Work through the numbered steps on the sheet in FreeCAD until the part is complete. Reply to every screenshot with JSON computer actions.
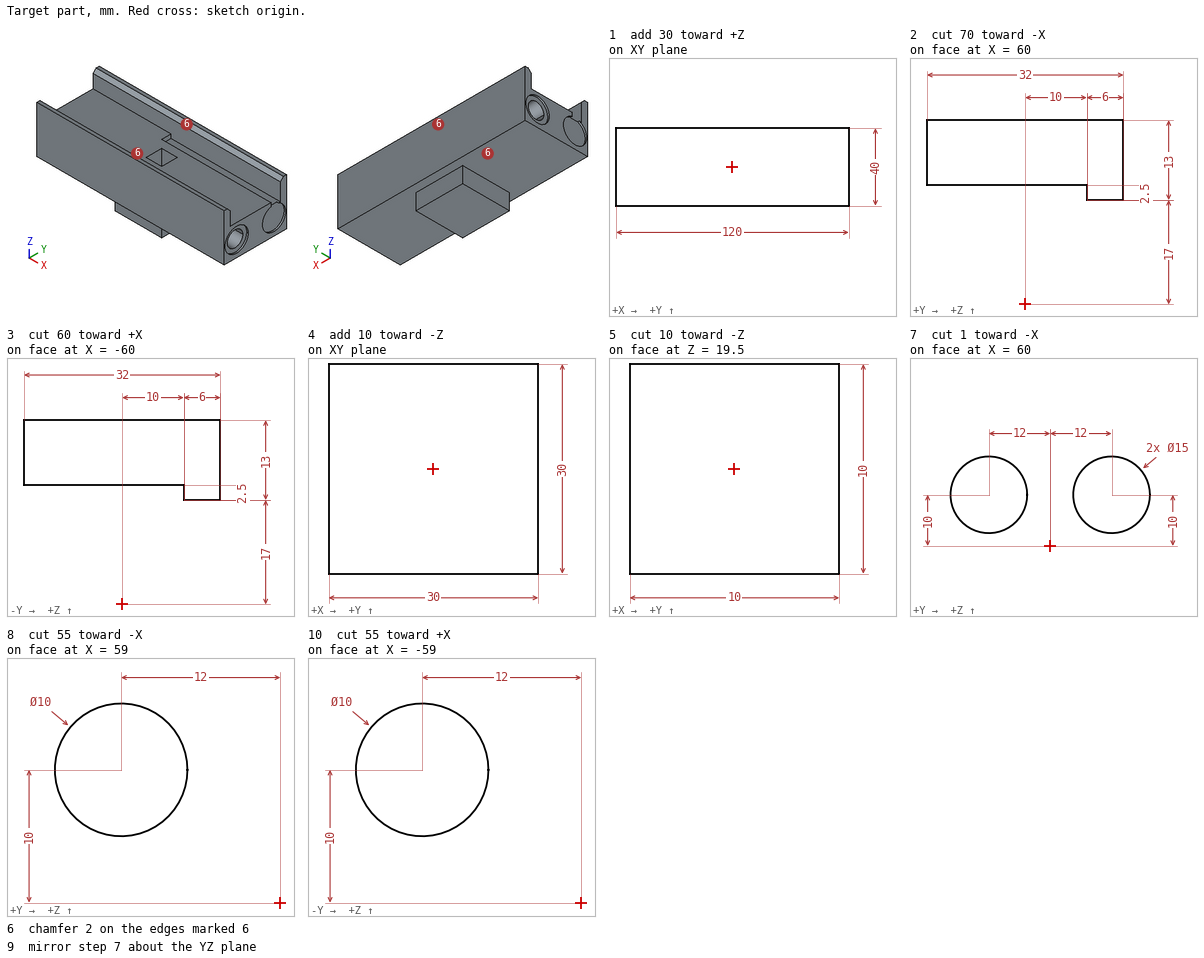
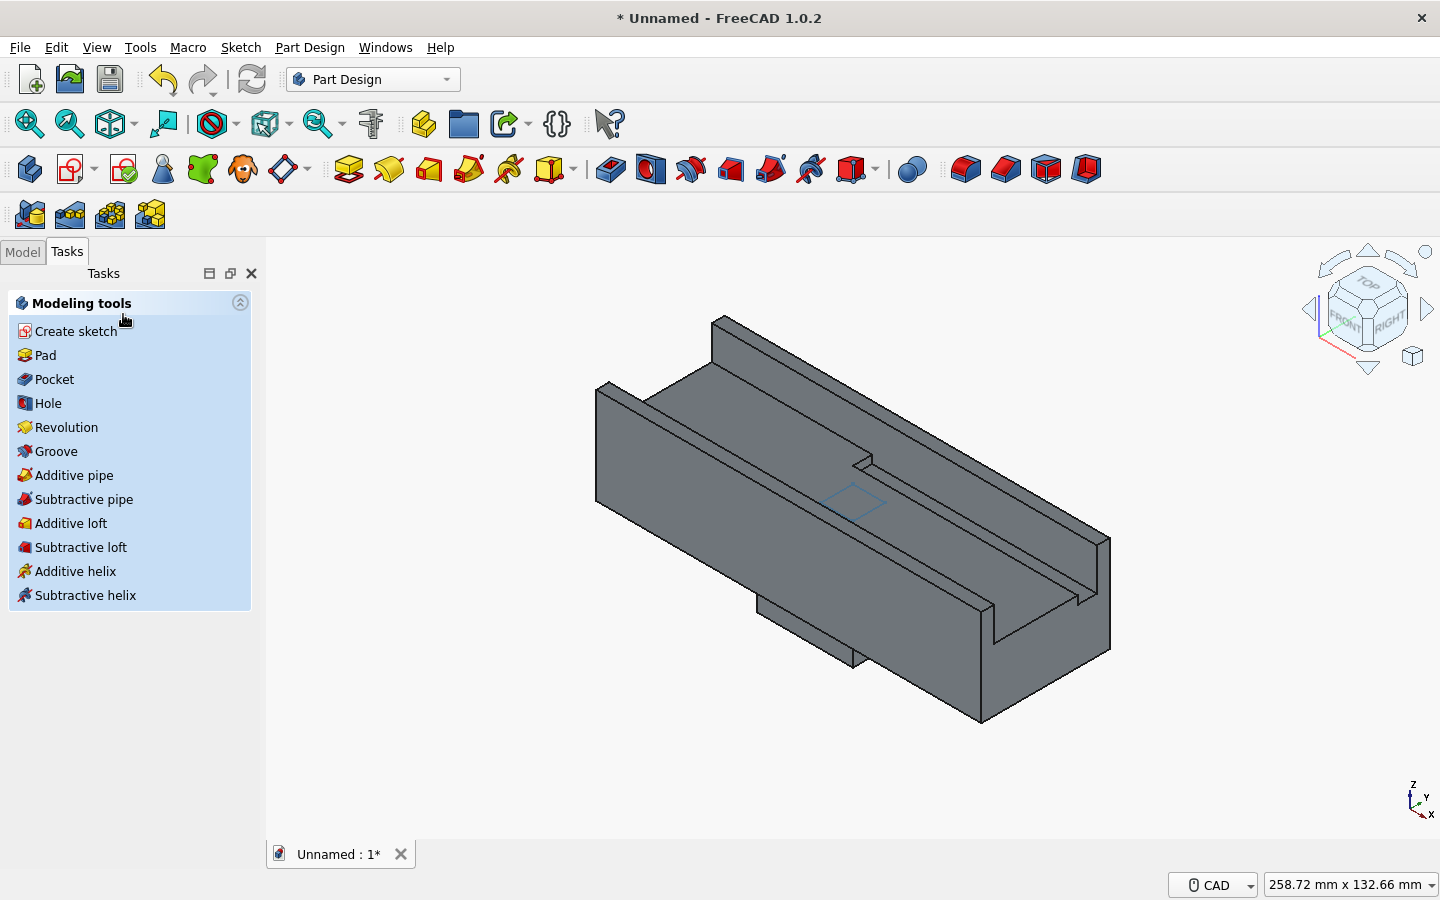
{"action": "left_click", "coordinate": [612, 170]}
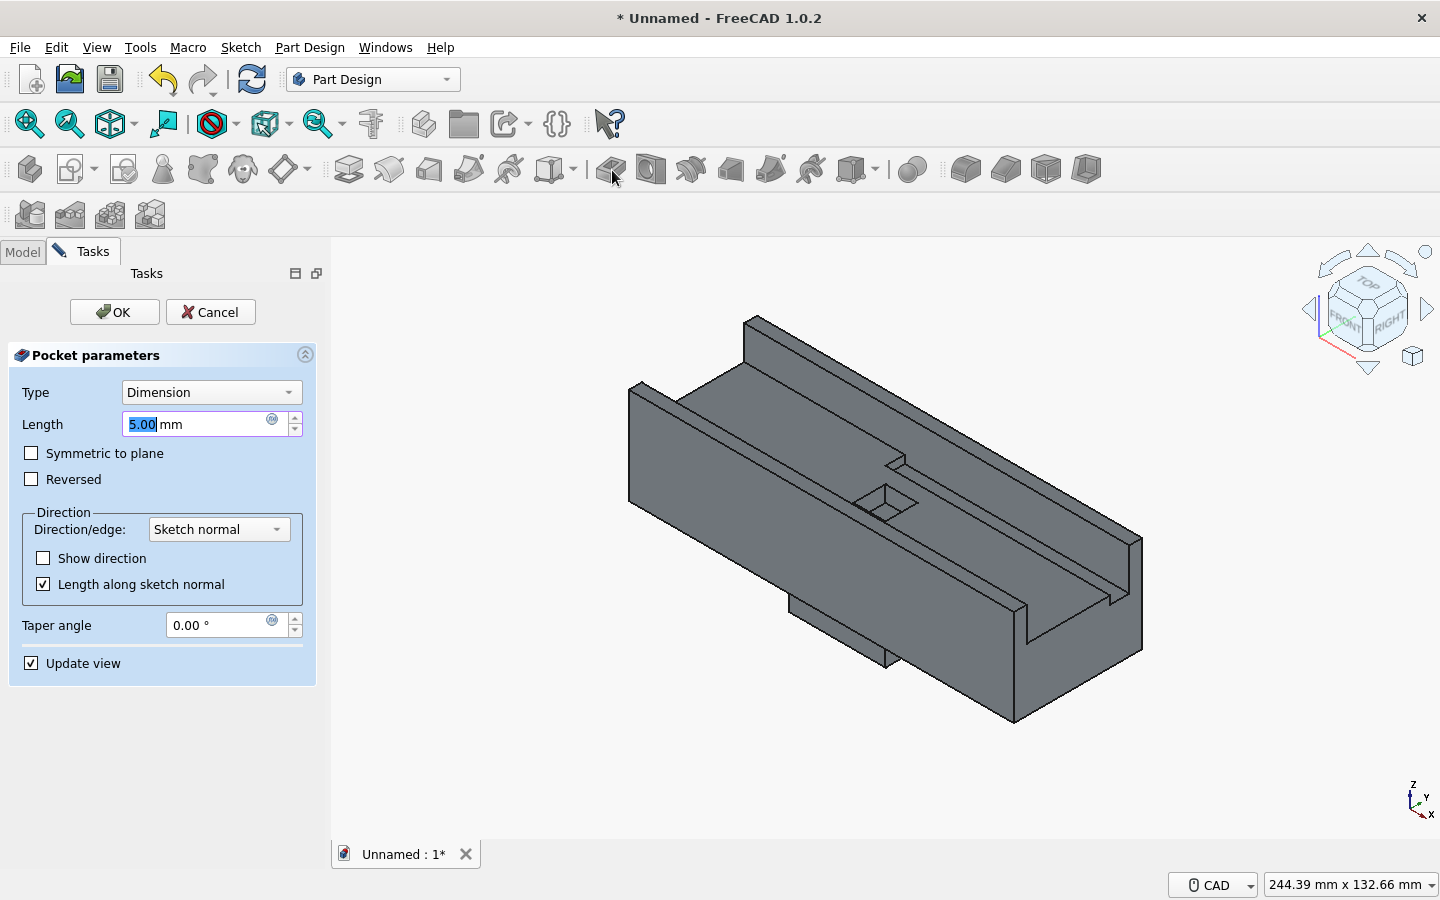
{"action": "type", "text": "10"}
{"action": "key", "text": "Tab"}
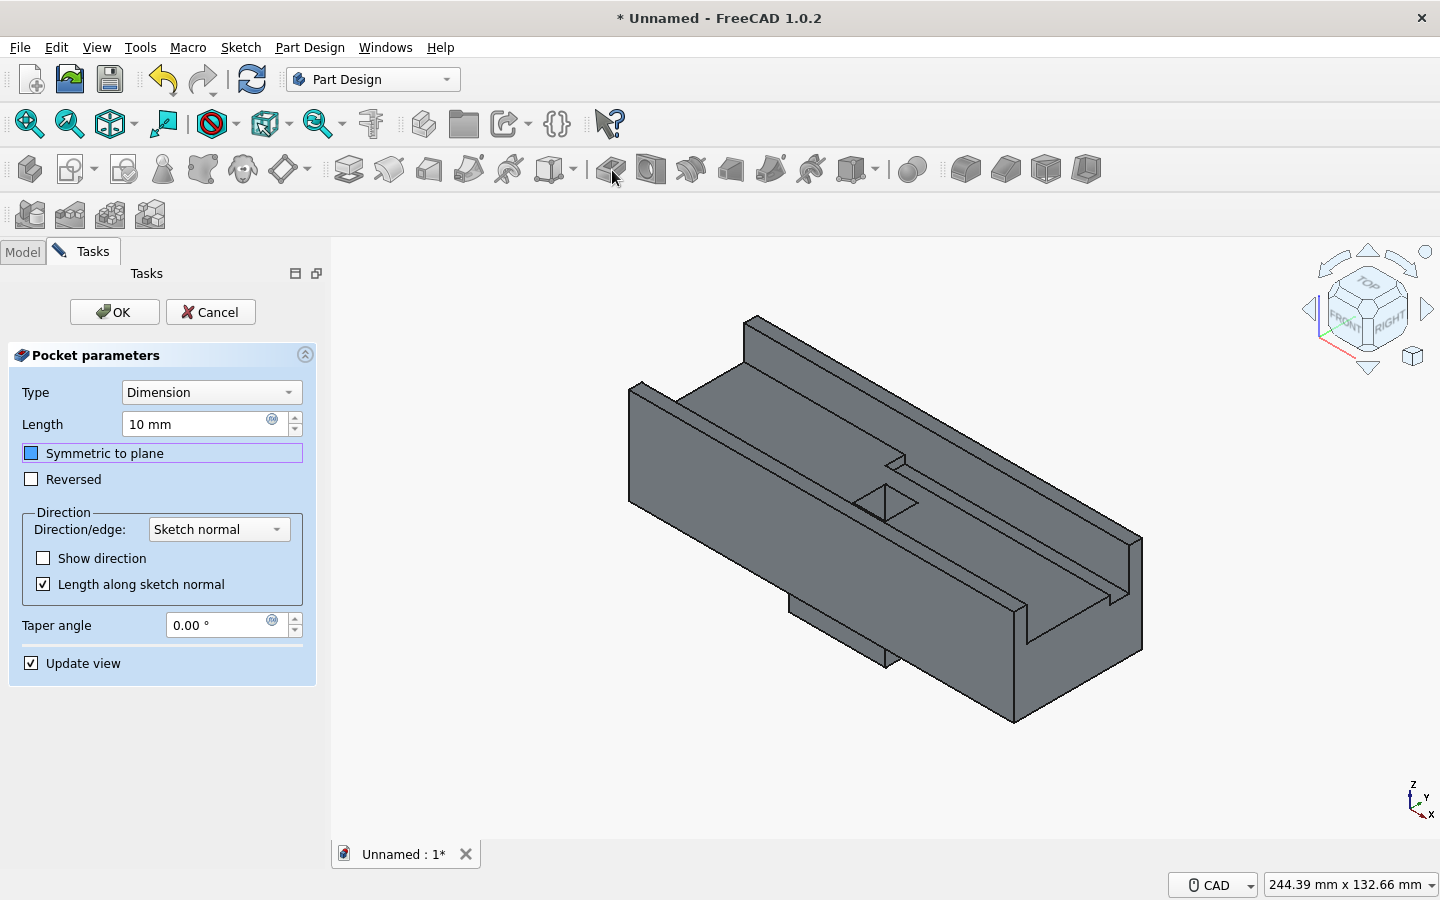
{"action": "left_click", "coordinate": [115, 312]}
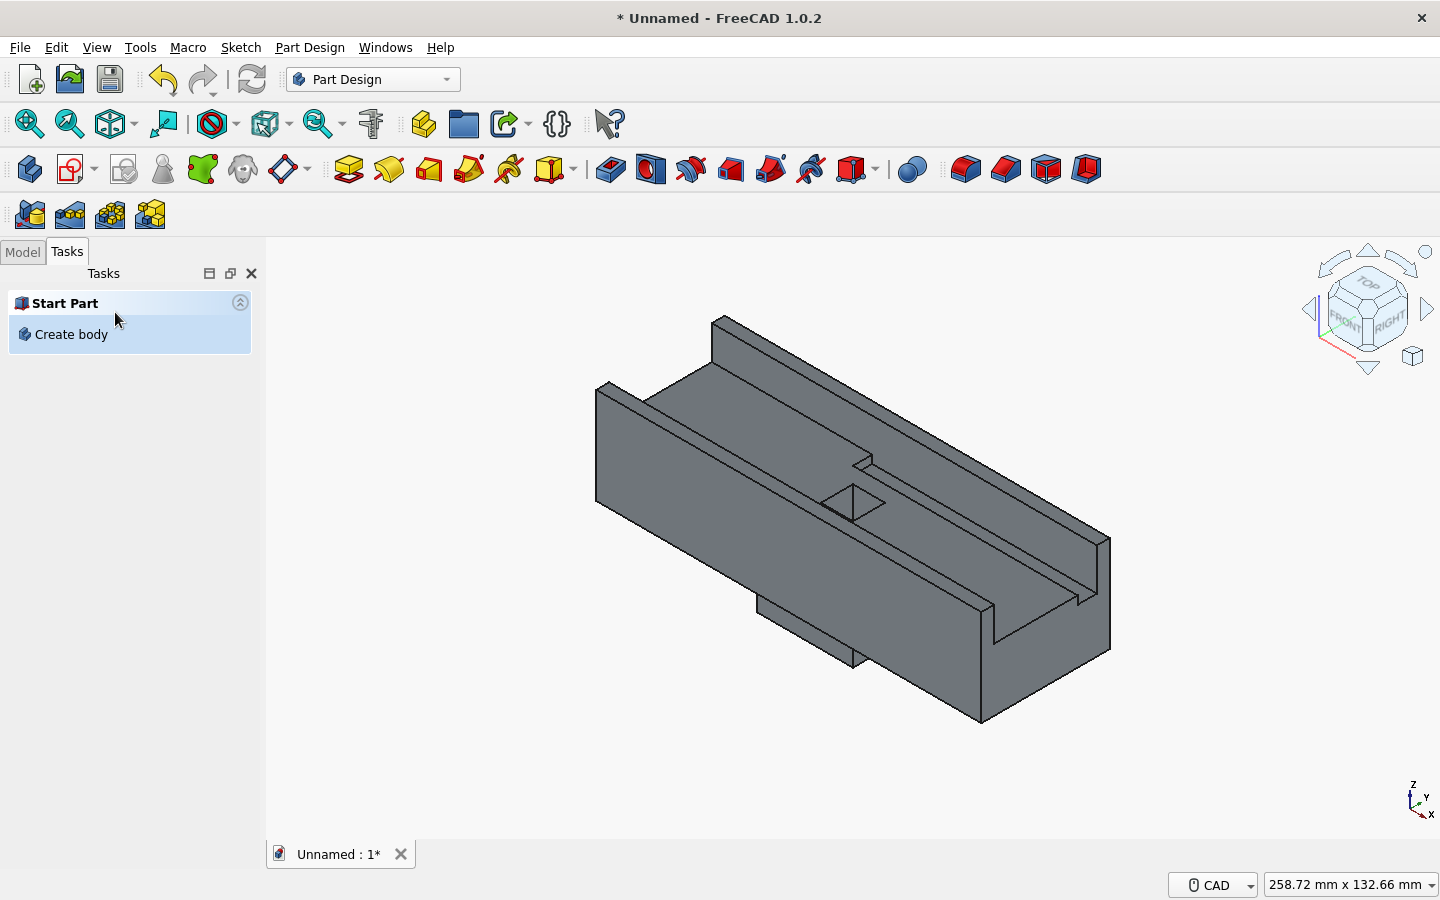
{"action": "left_click", "coordinate": [904, 433]}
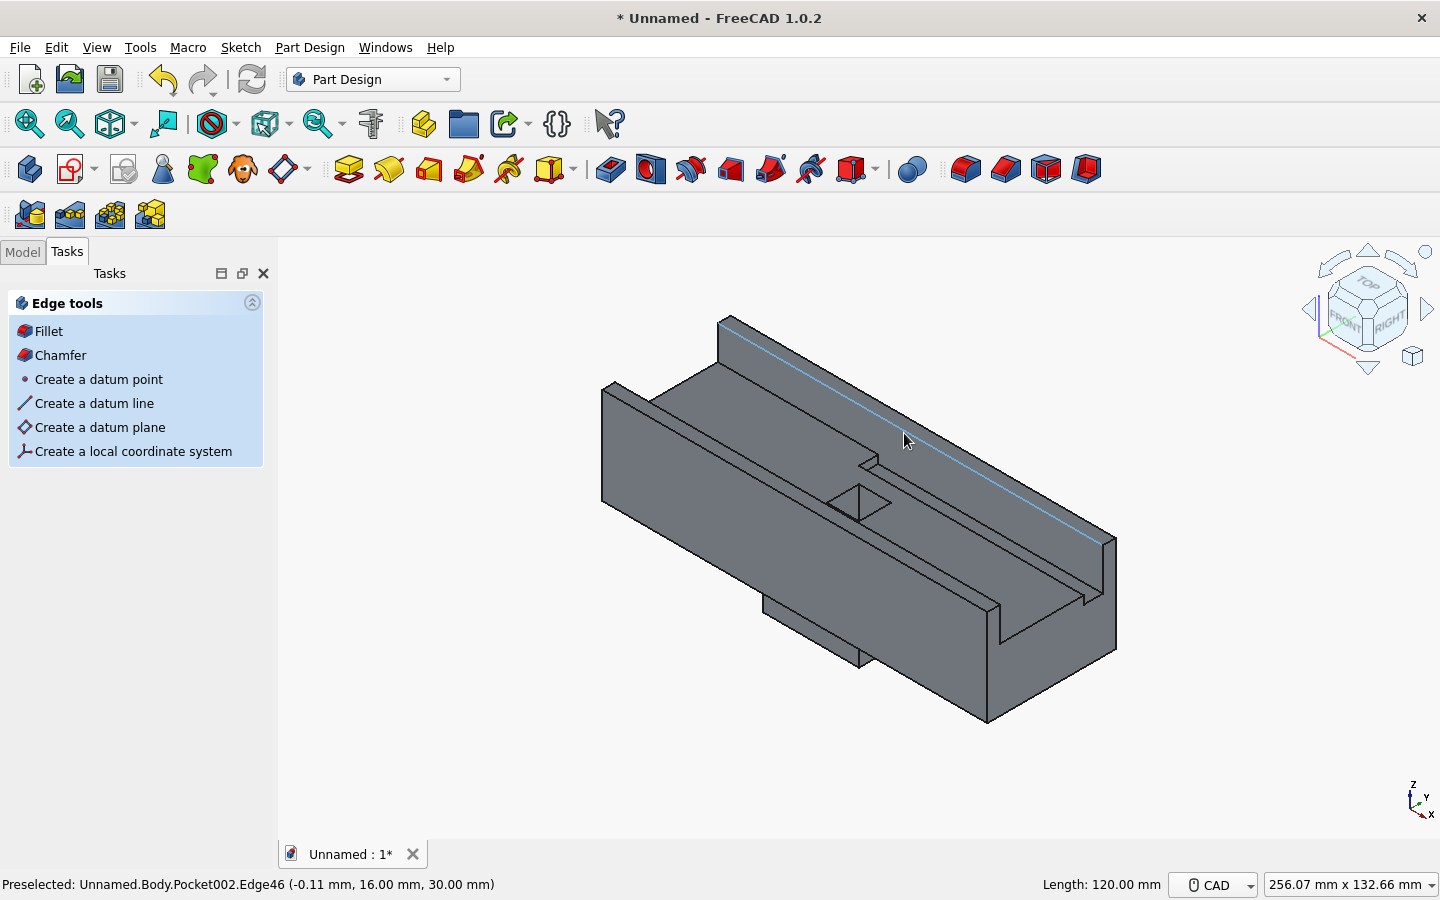
{"action": "key", "text": "2"}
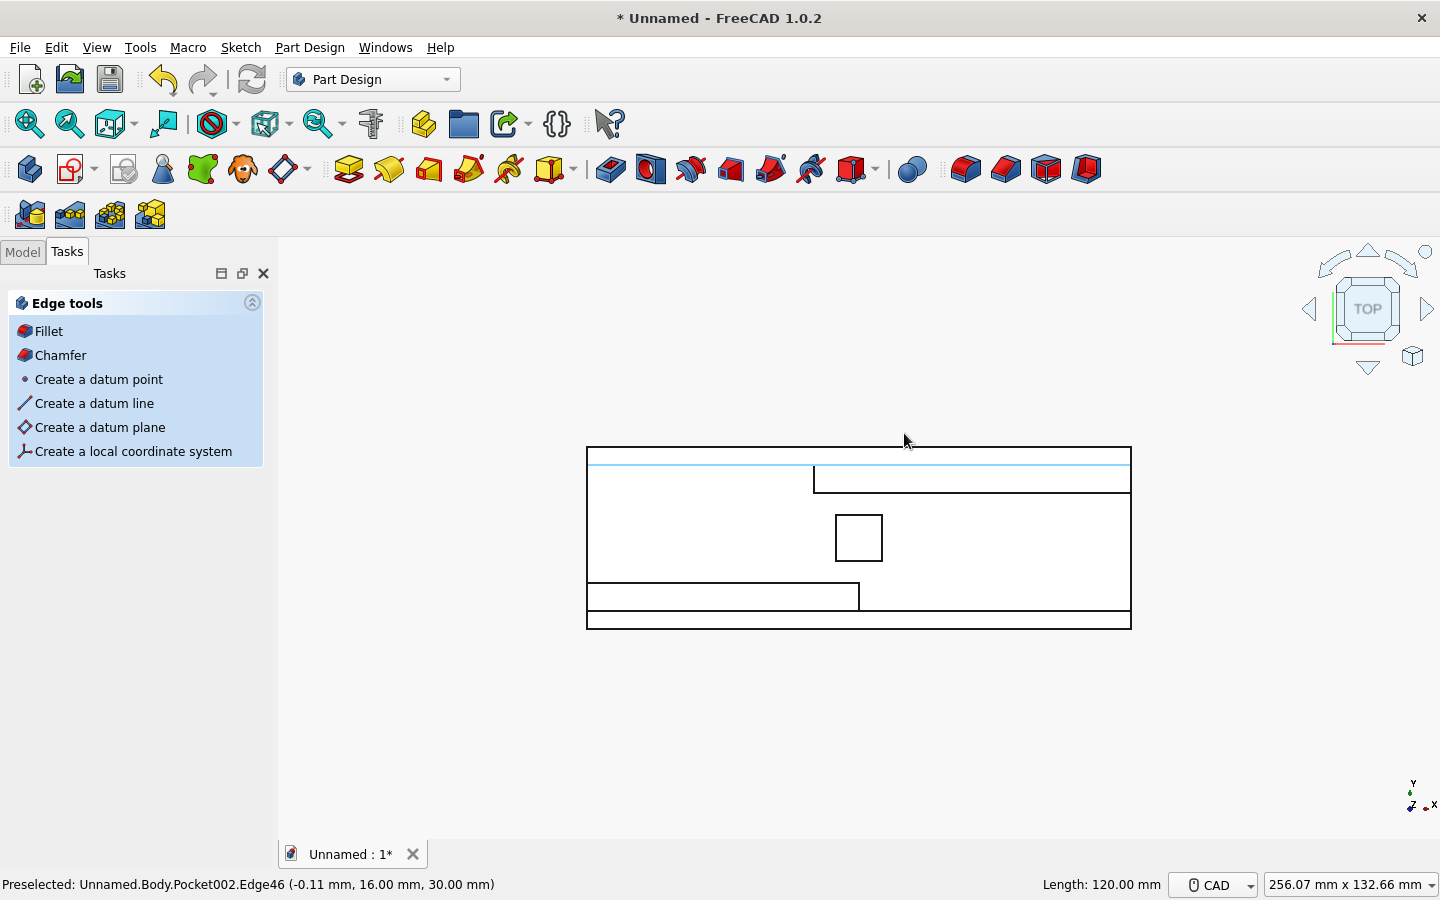
{"action": "left_click", "coordinate": [859, 610], "text": "ctrl"}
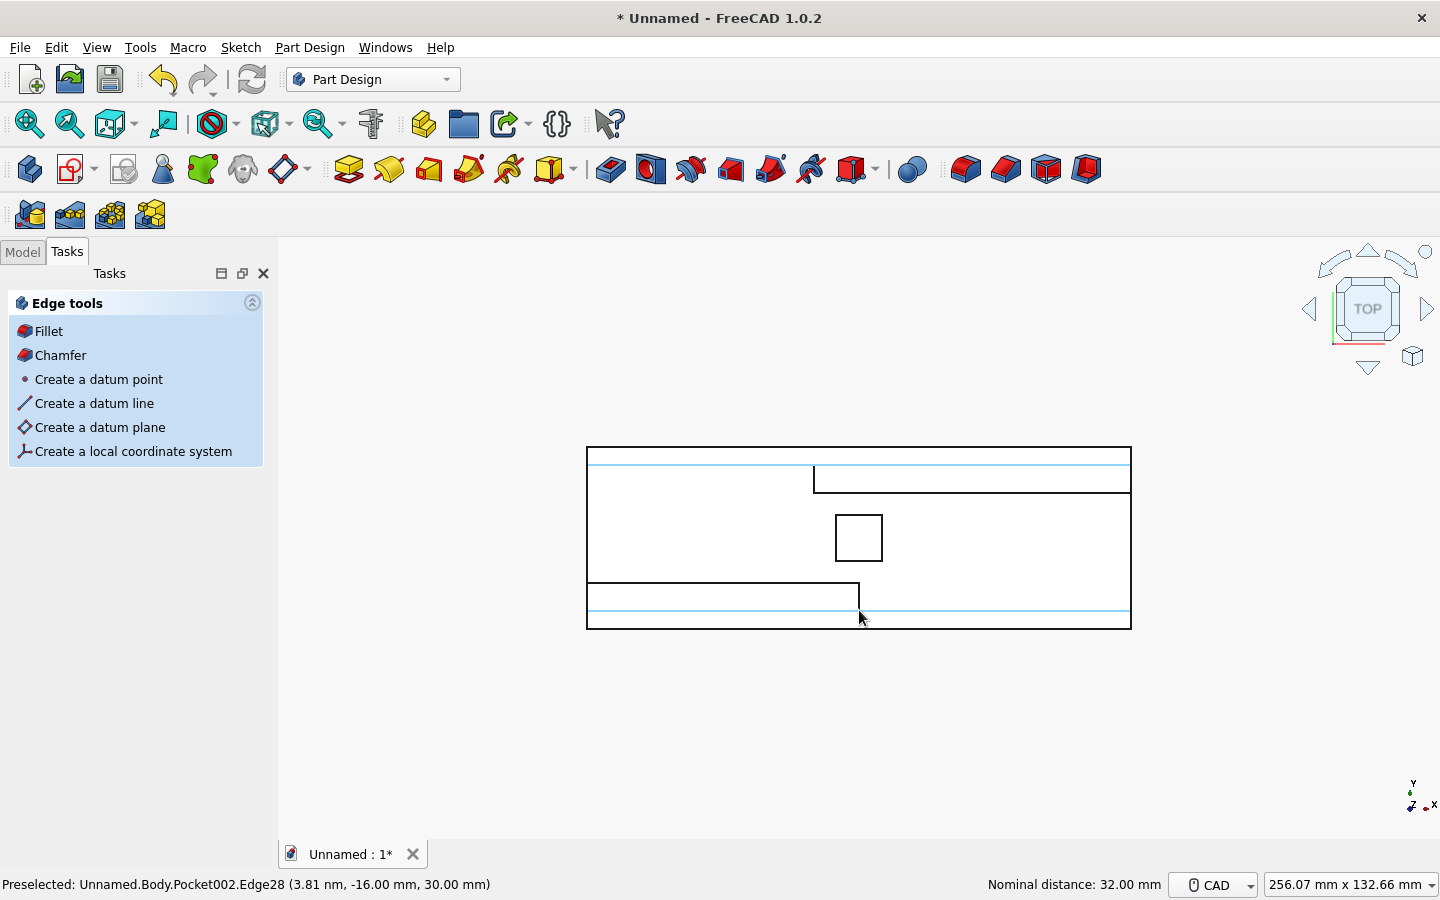
{"action": "left_click", "coordinate": [1006, 170]}